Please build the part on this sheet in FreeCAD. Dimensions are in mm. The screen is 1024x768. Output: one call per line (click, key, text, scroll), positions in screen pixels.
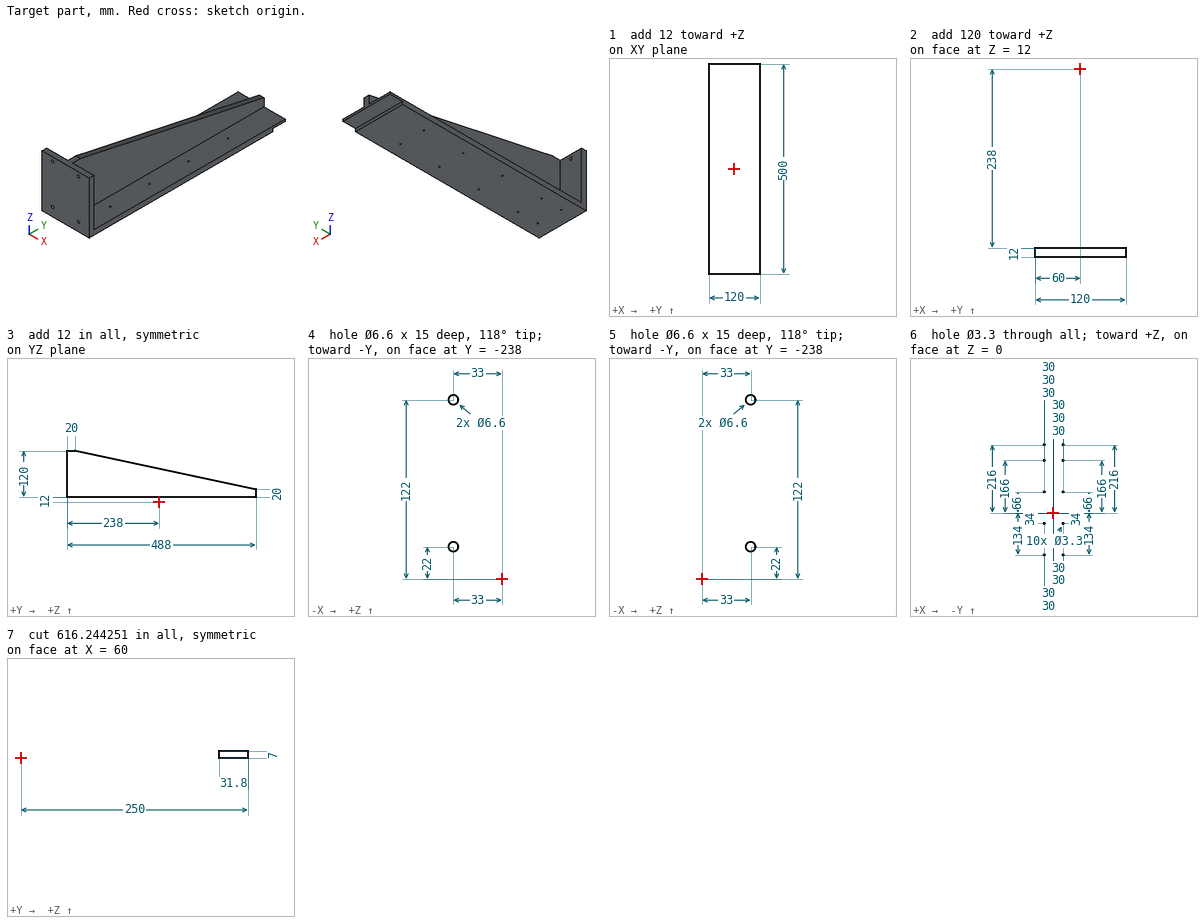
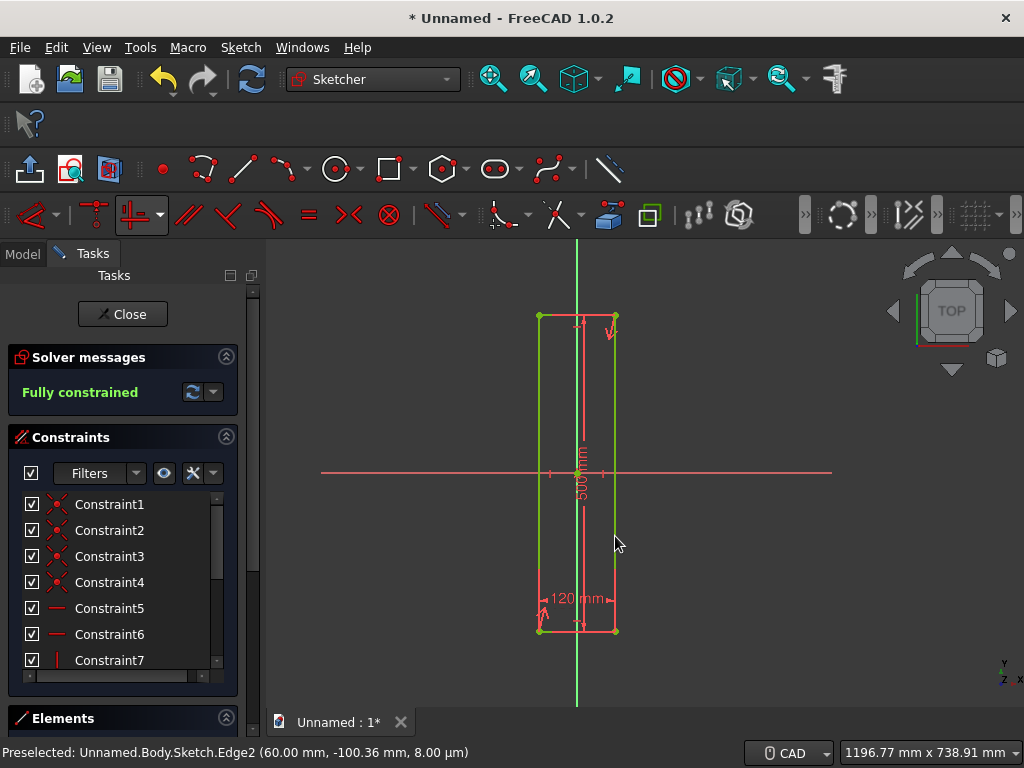
click(123, 314)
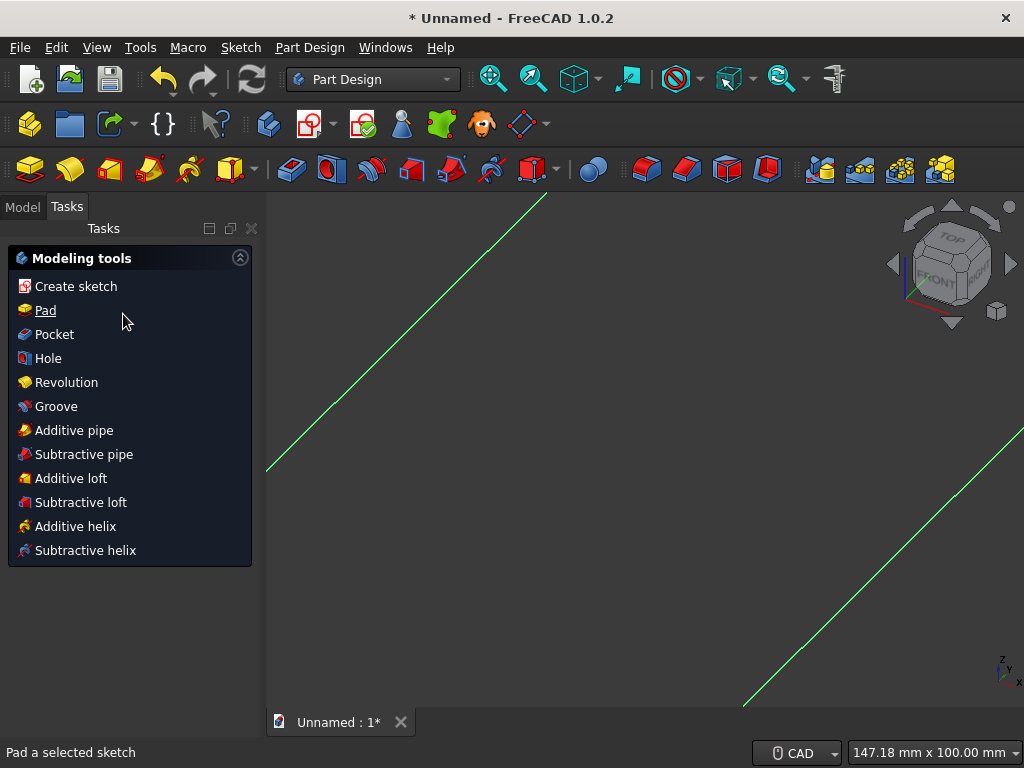
click(30, 170)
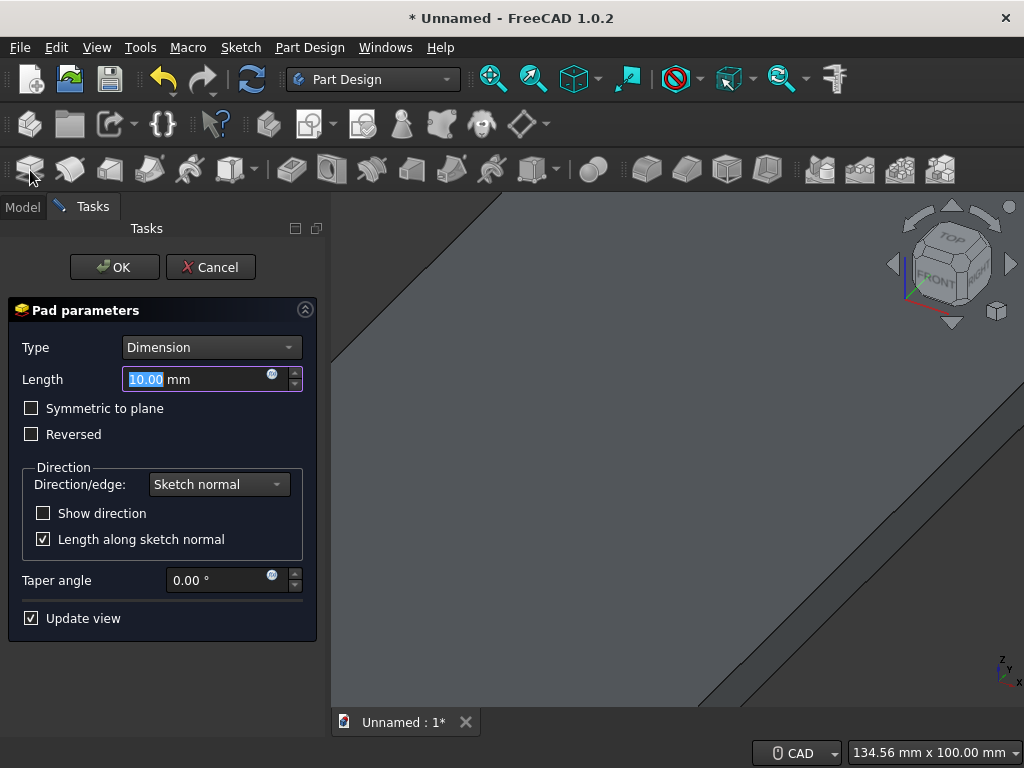
text(12)
key(Tab)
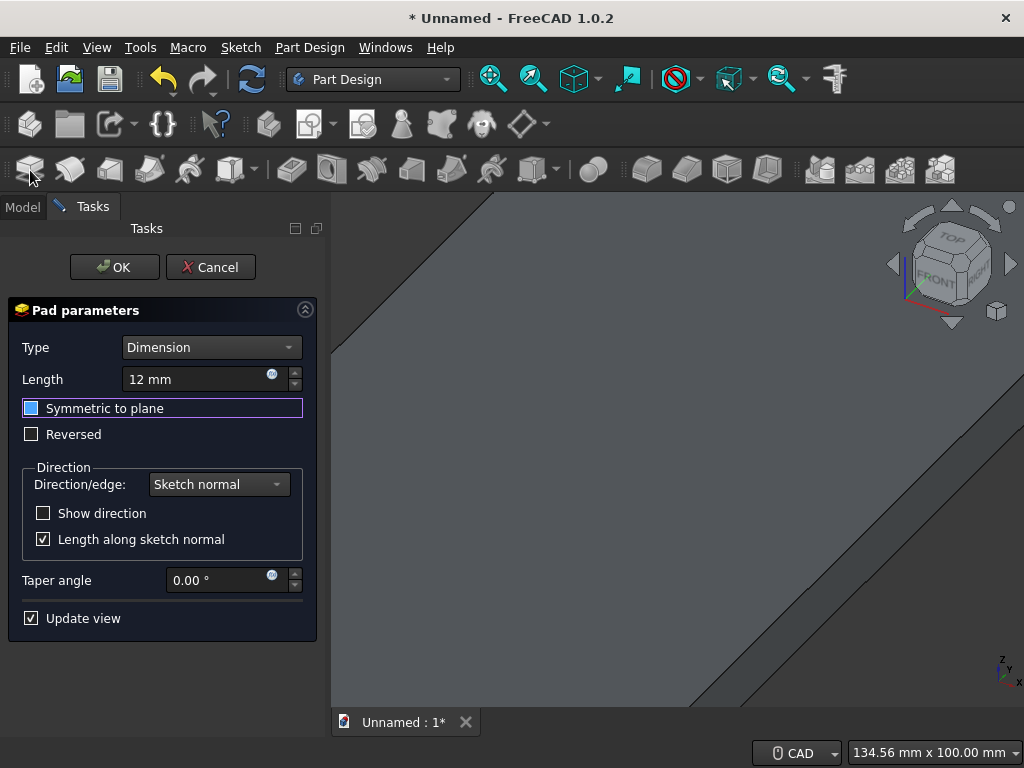
click(115, 267)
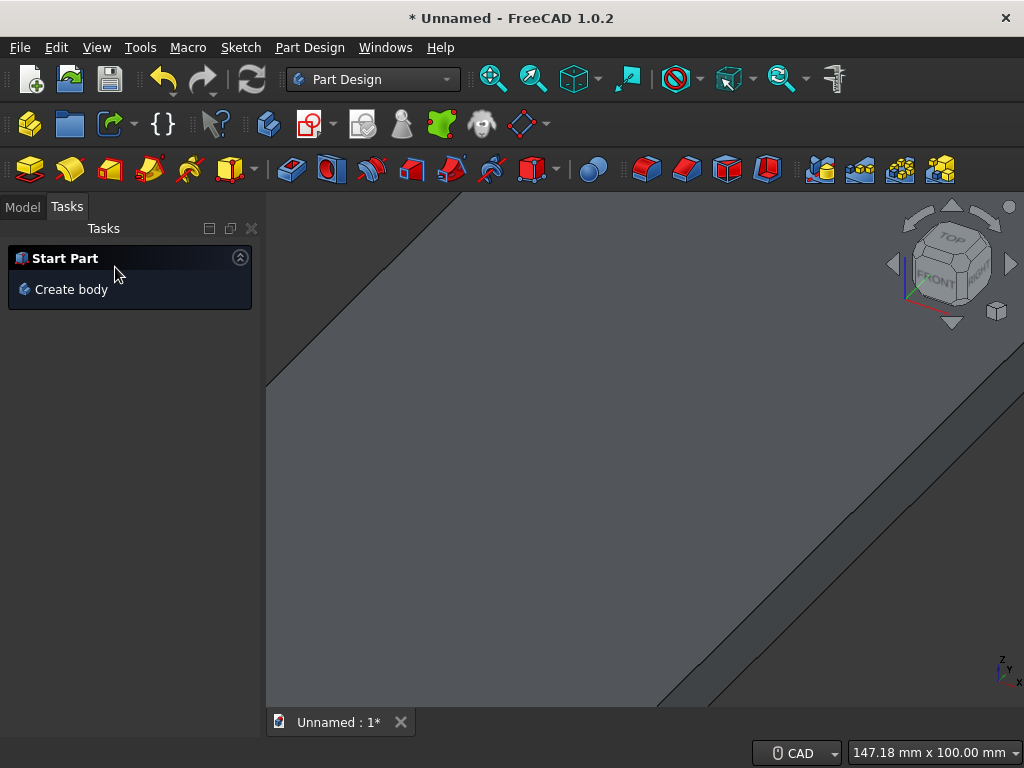
click(494, 80)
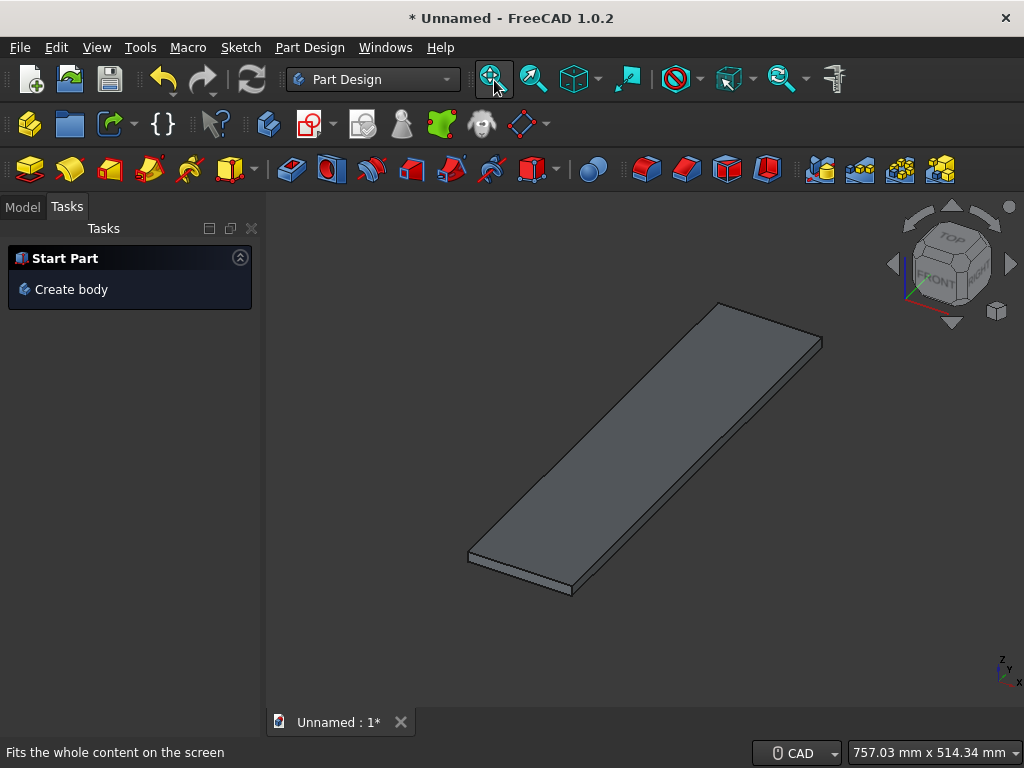
click(717, 373)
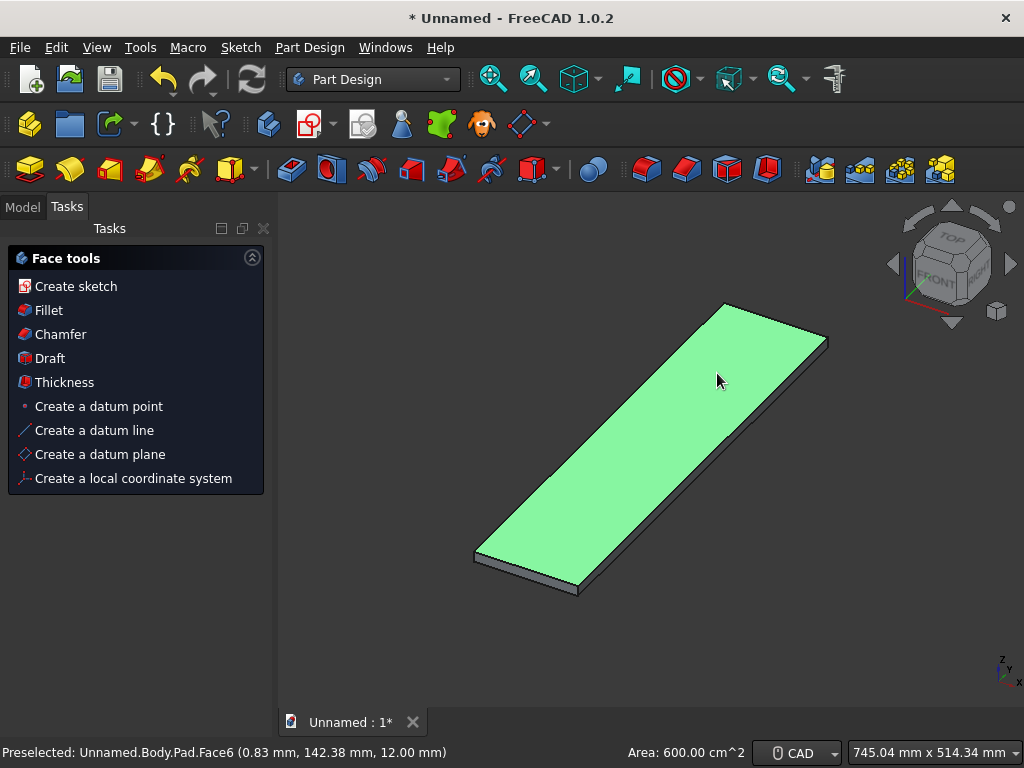
click(310, 124)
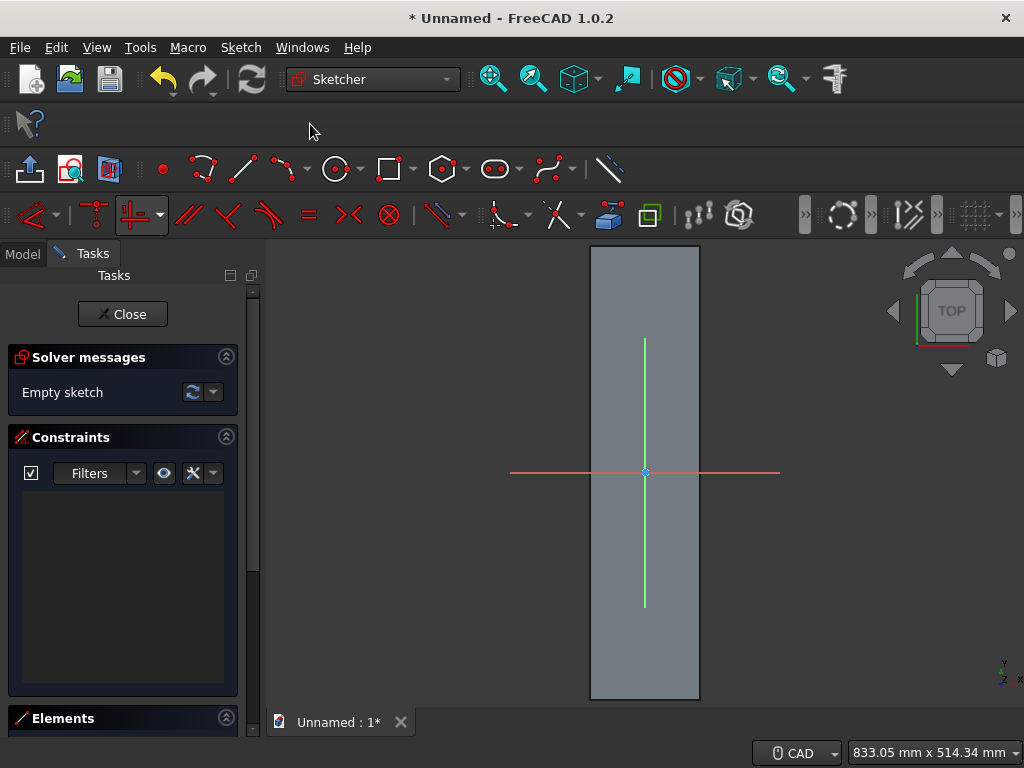
scroll(294, 267, down, 1)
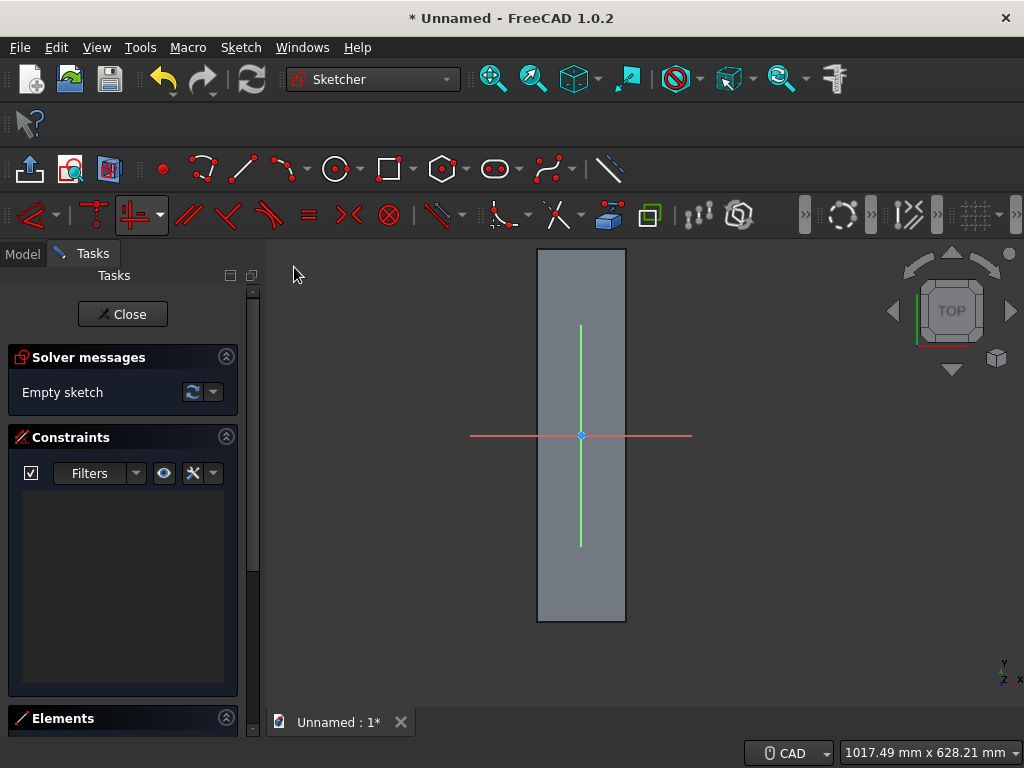
scroll(591, 642, up, 2)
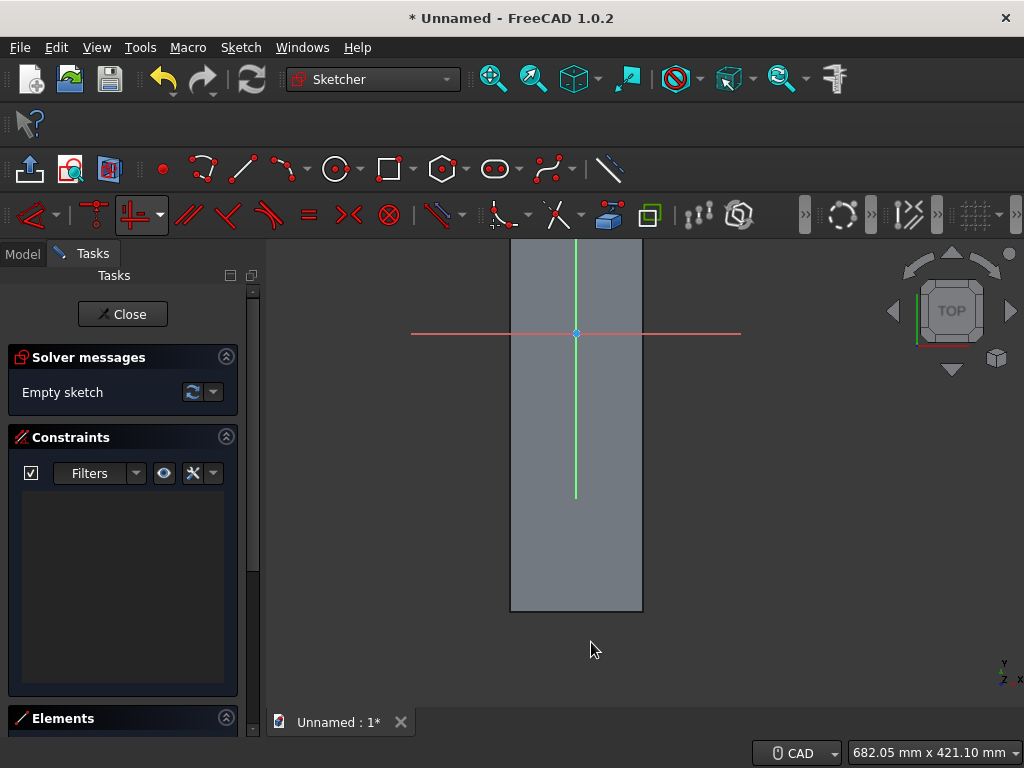
click(390, 170)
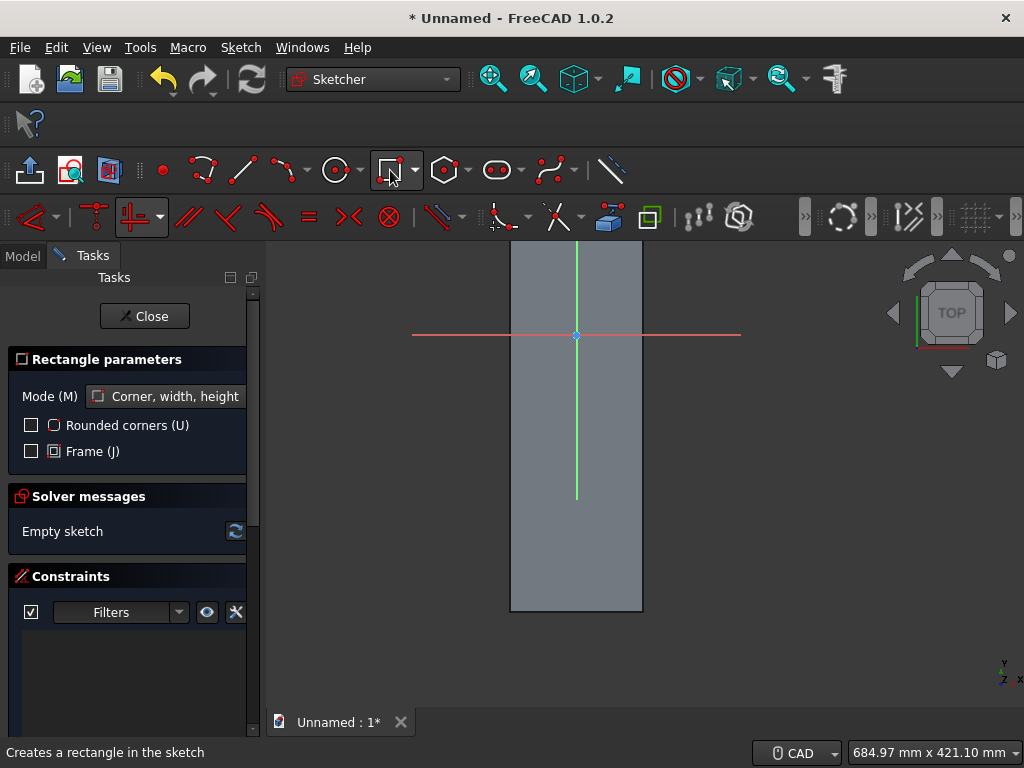
click(510, 599)
click(643, 612)
key(Escape)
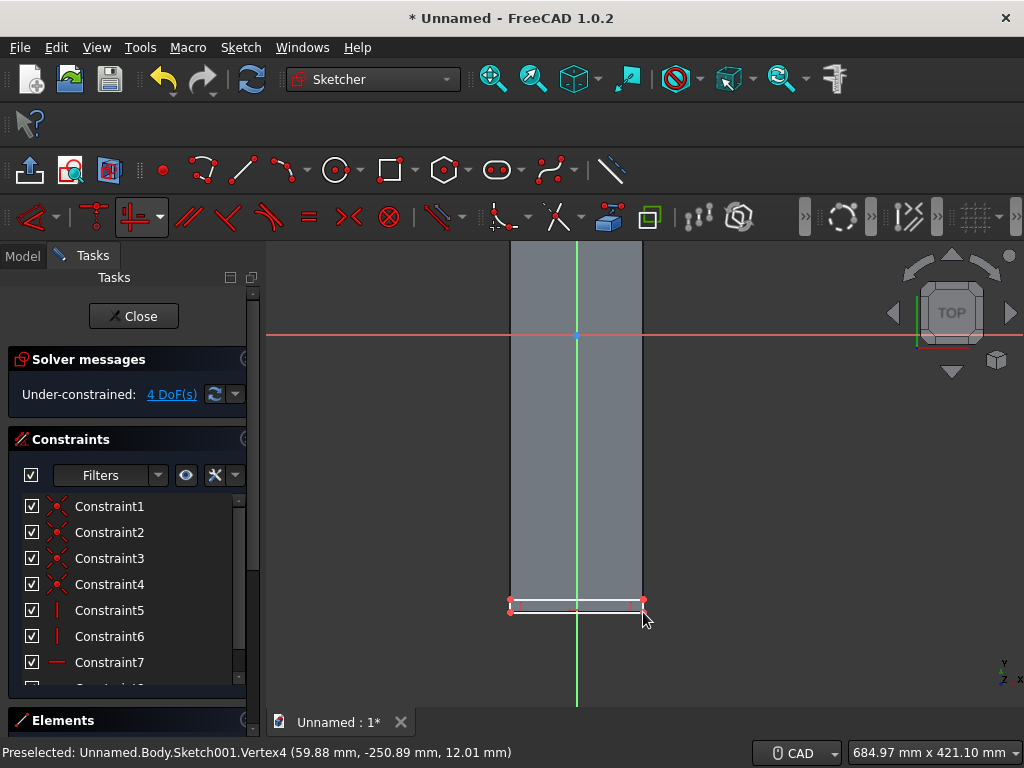
scroll(510, 607, up, 6)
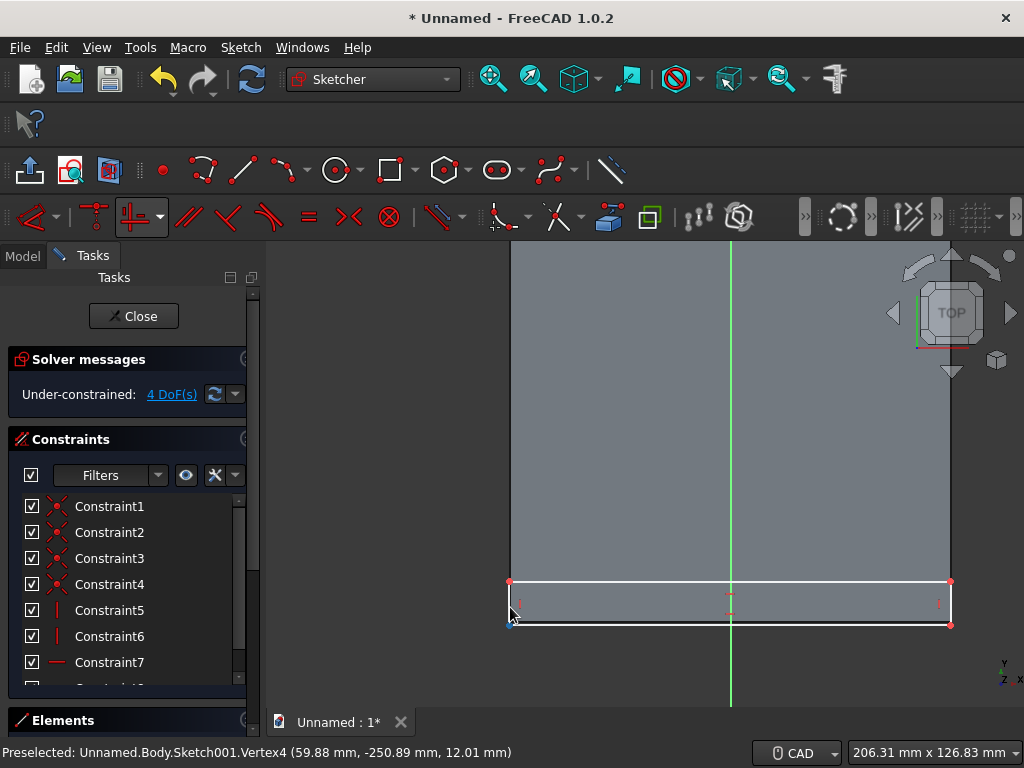
click(509, 604)